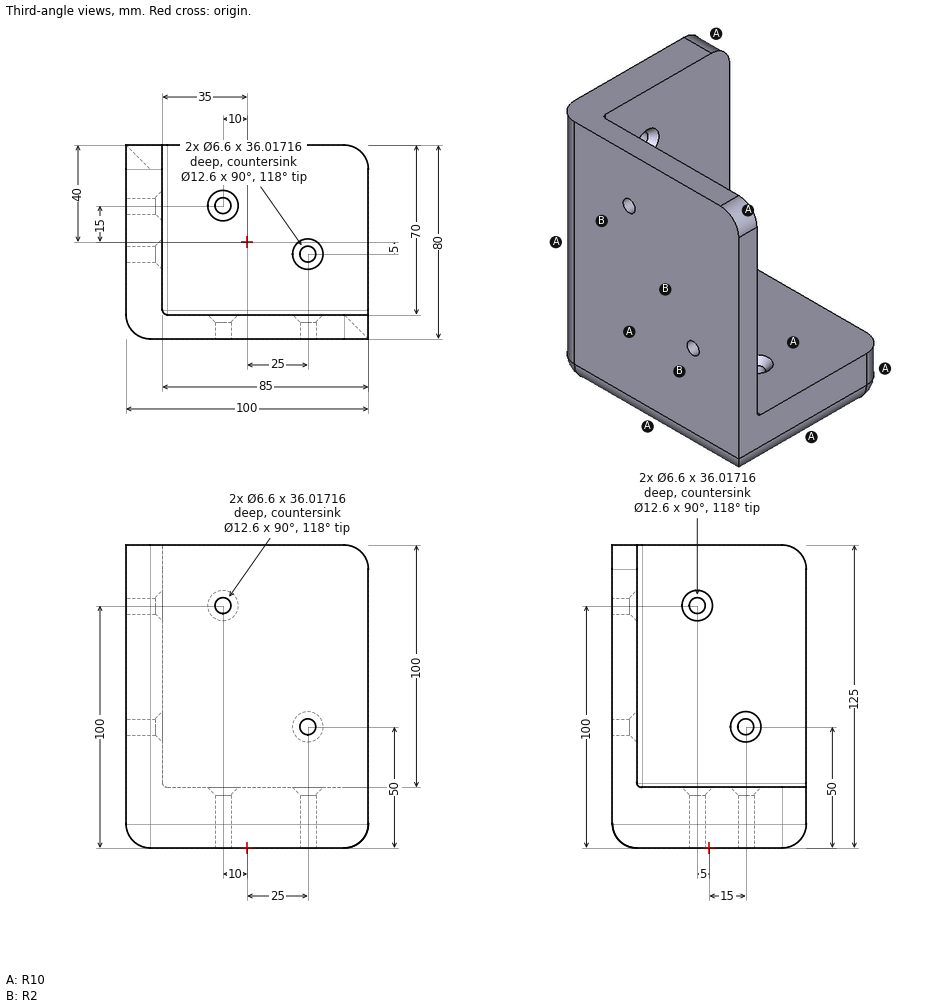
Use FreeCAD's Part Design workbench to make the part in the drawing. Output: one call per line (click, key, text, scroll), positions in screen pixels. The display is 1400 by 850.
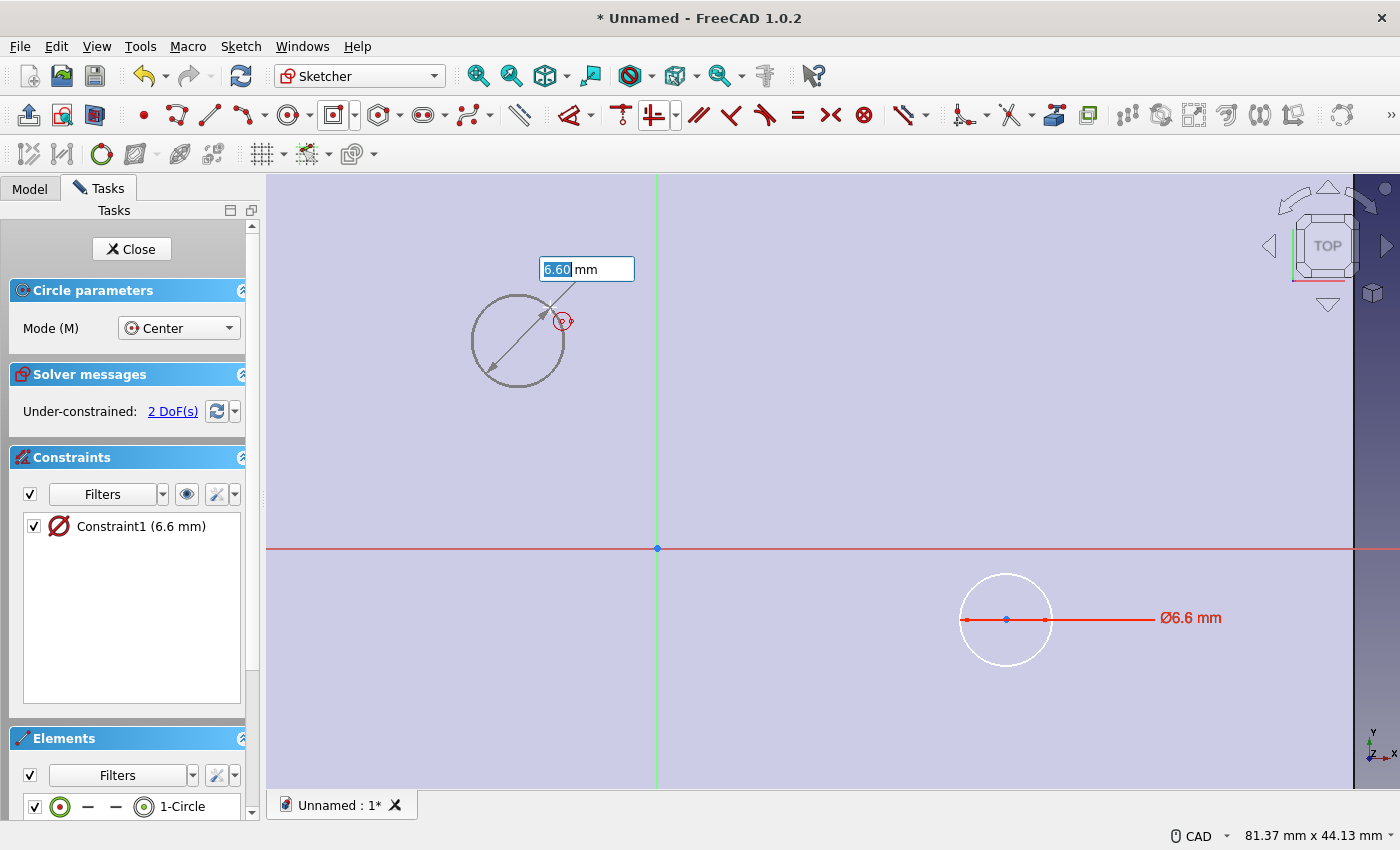
text(6.6)
key(Return)
key(Escape)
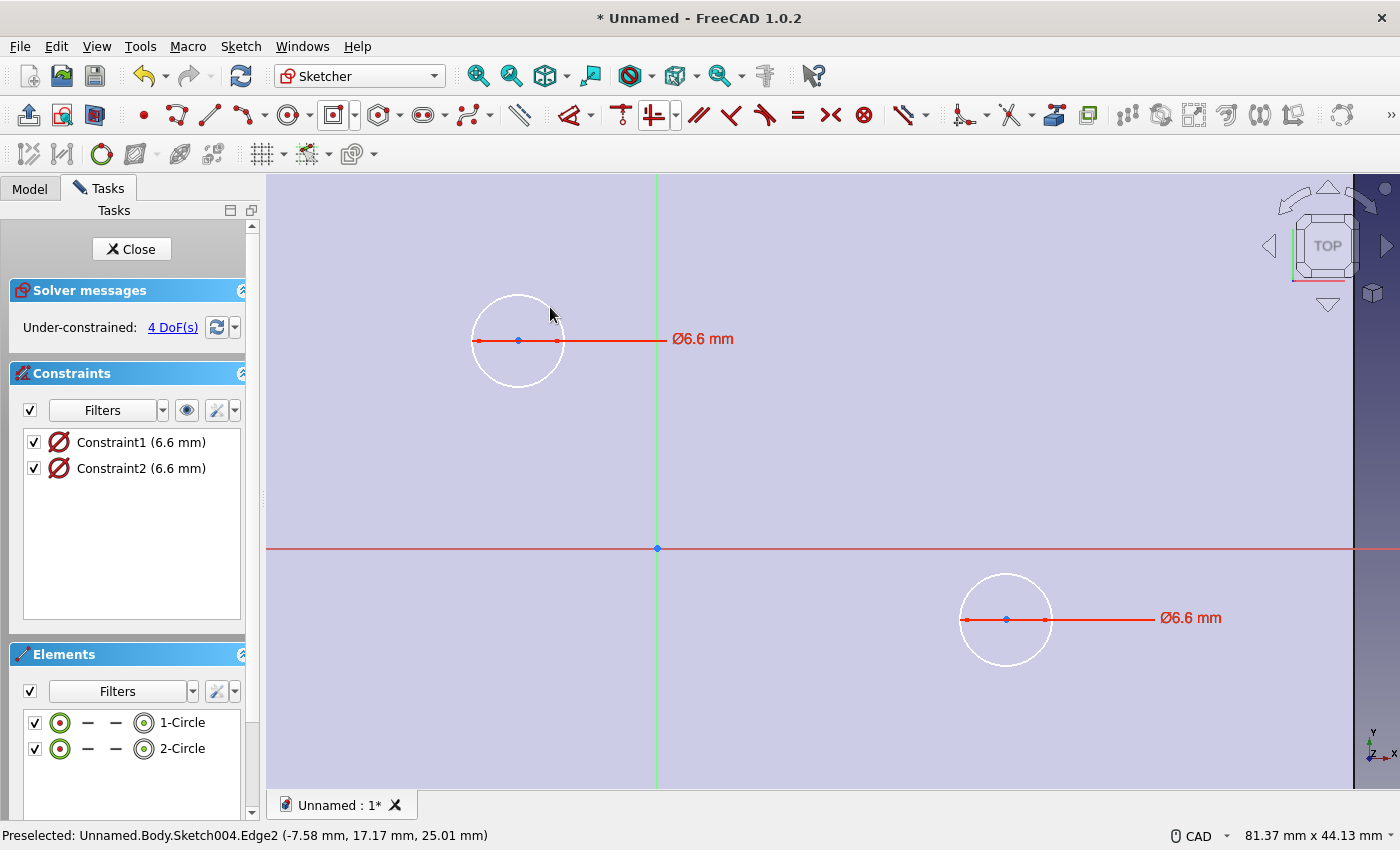
key(d)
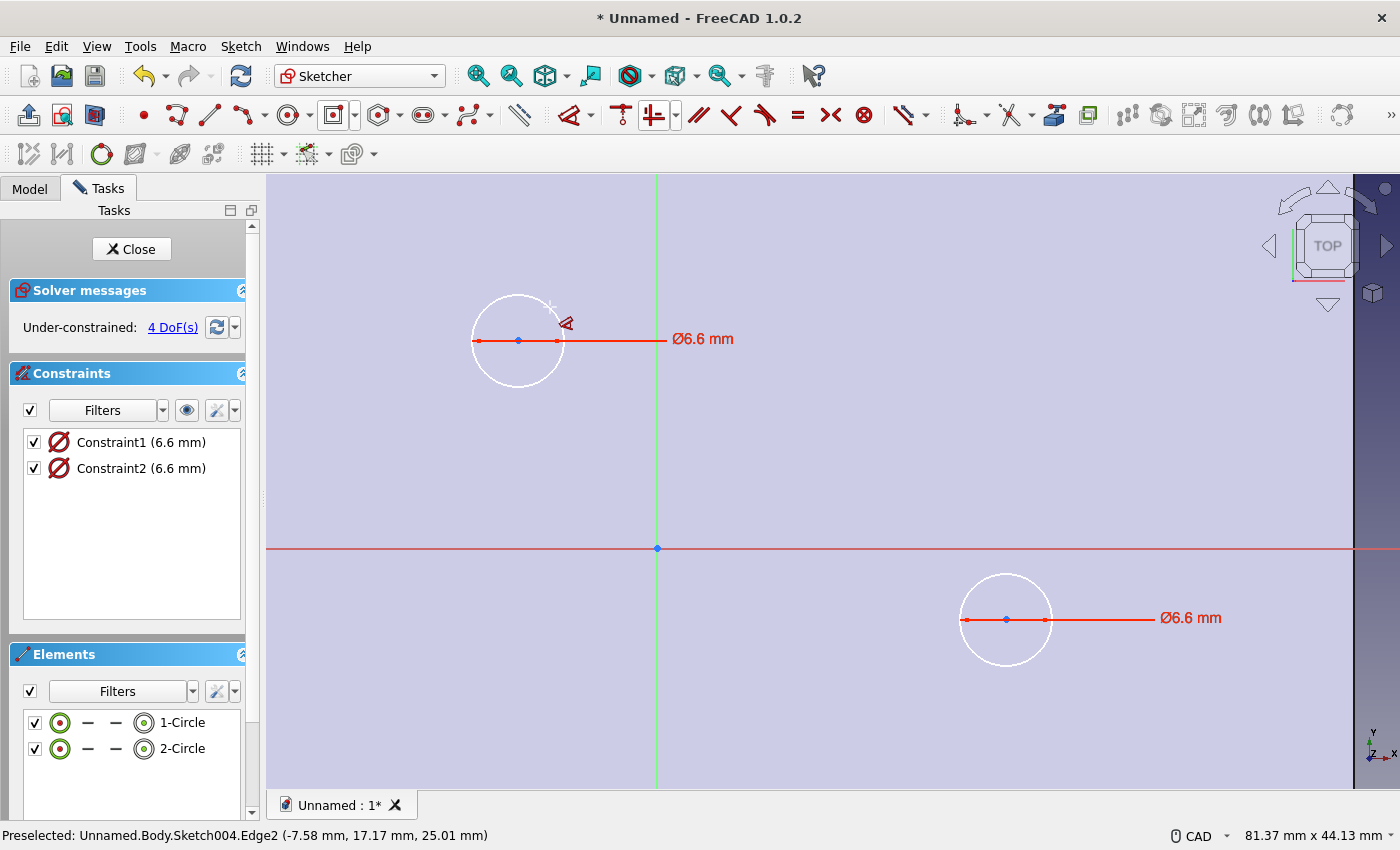
click(1006, 620)
click(1040, 568)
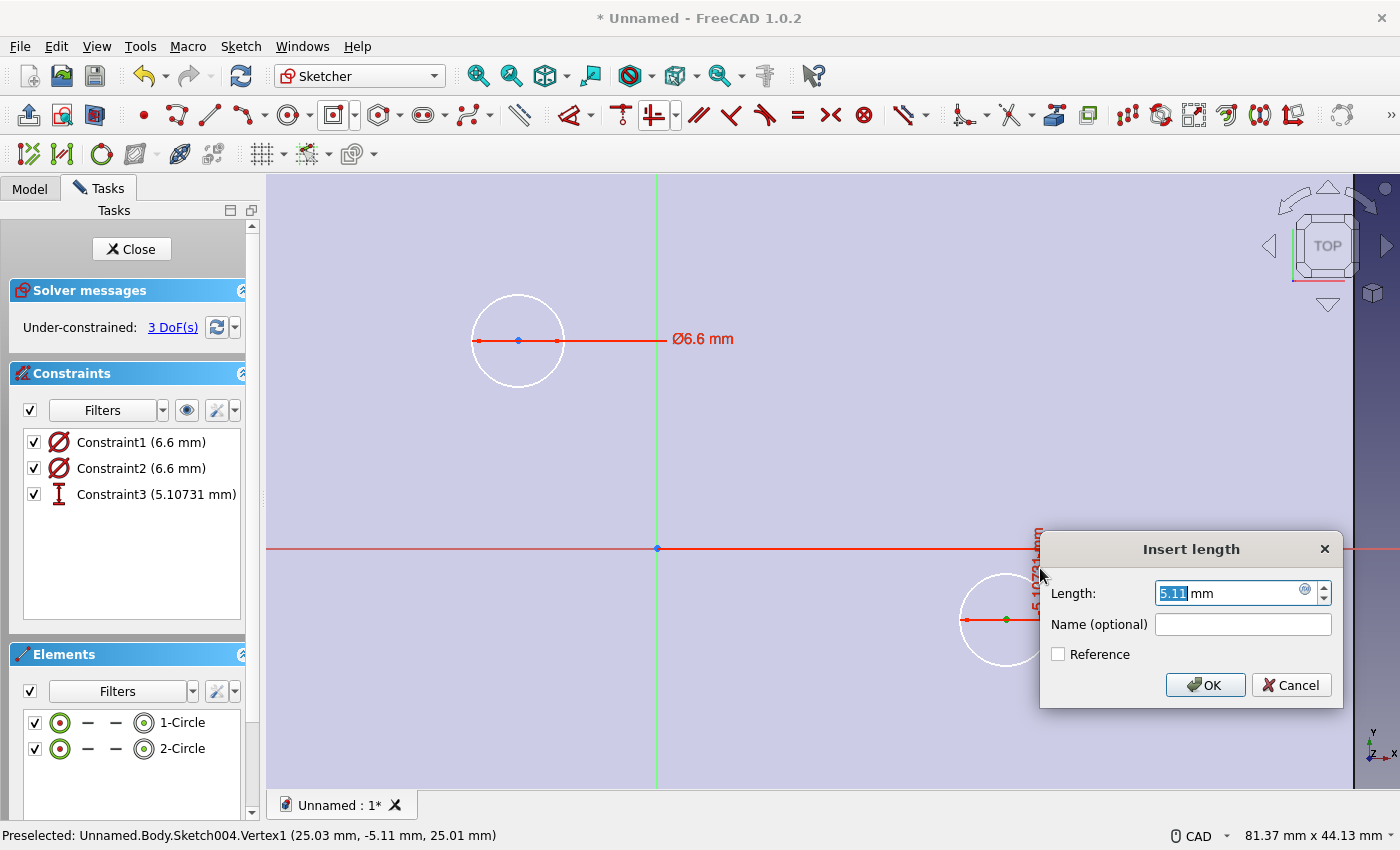
text(5)
key(Return)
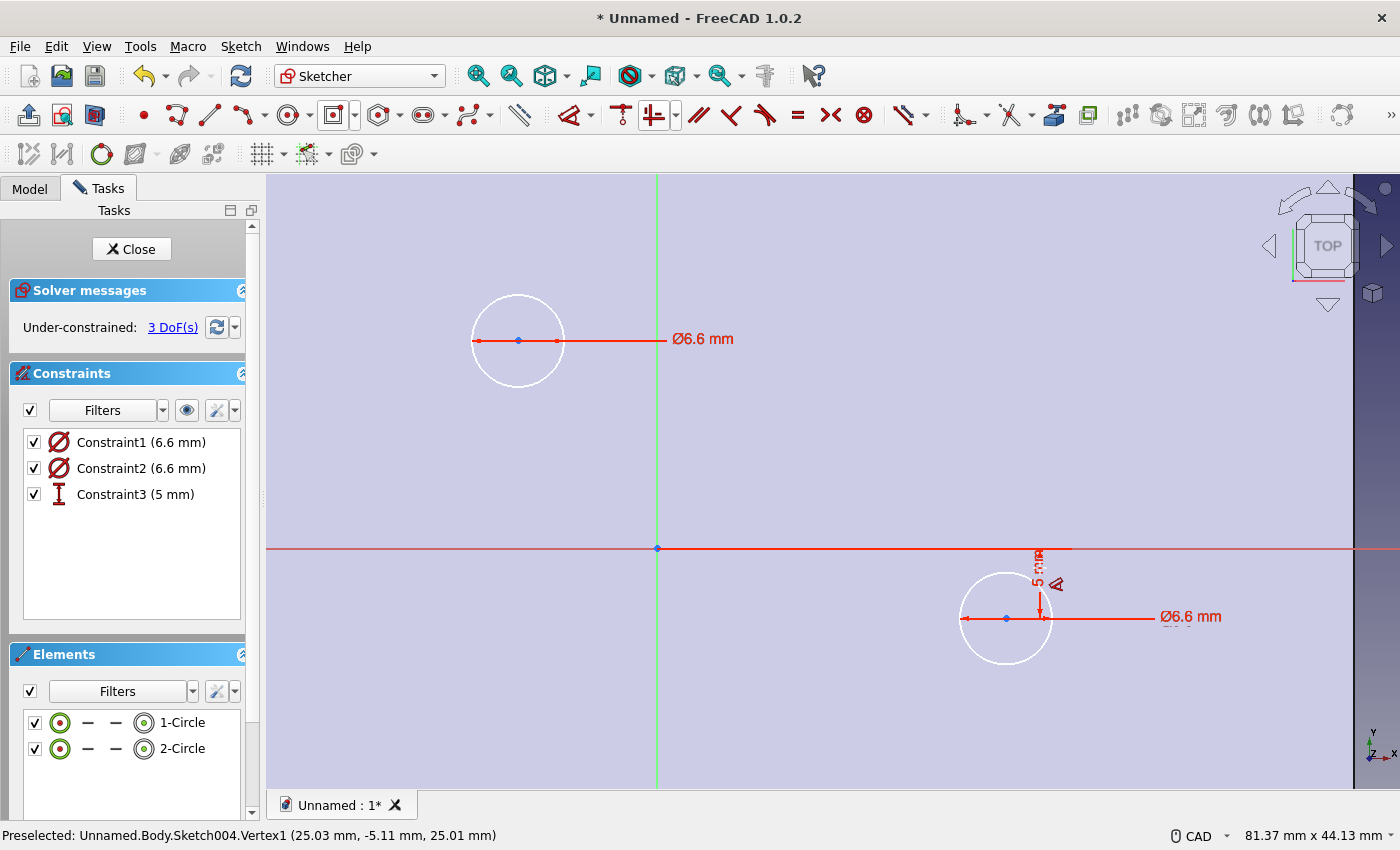
click(1006, 619)
click(832, 653)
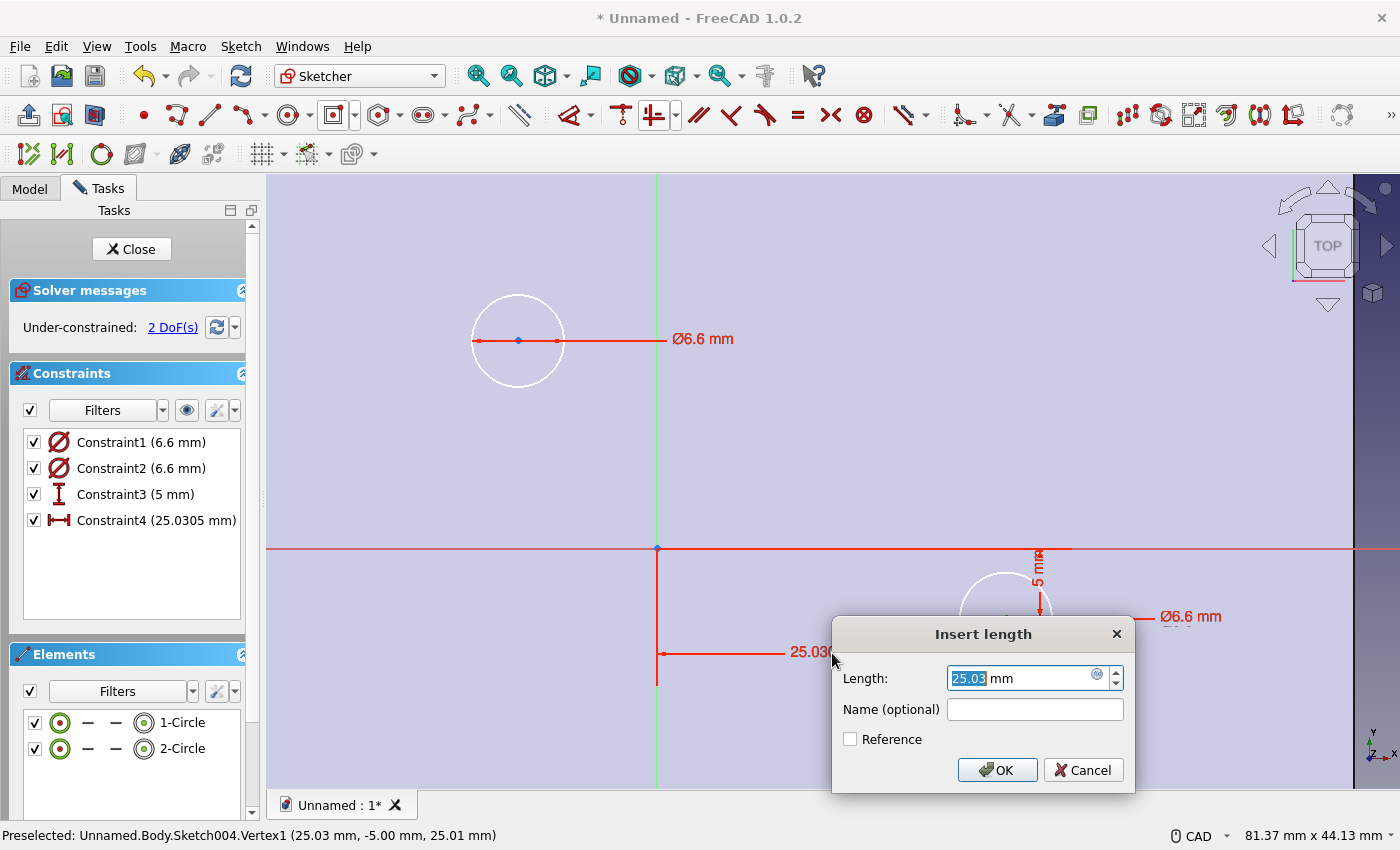
text(25)
key(Return)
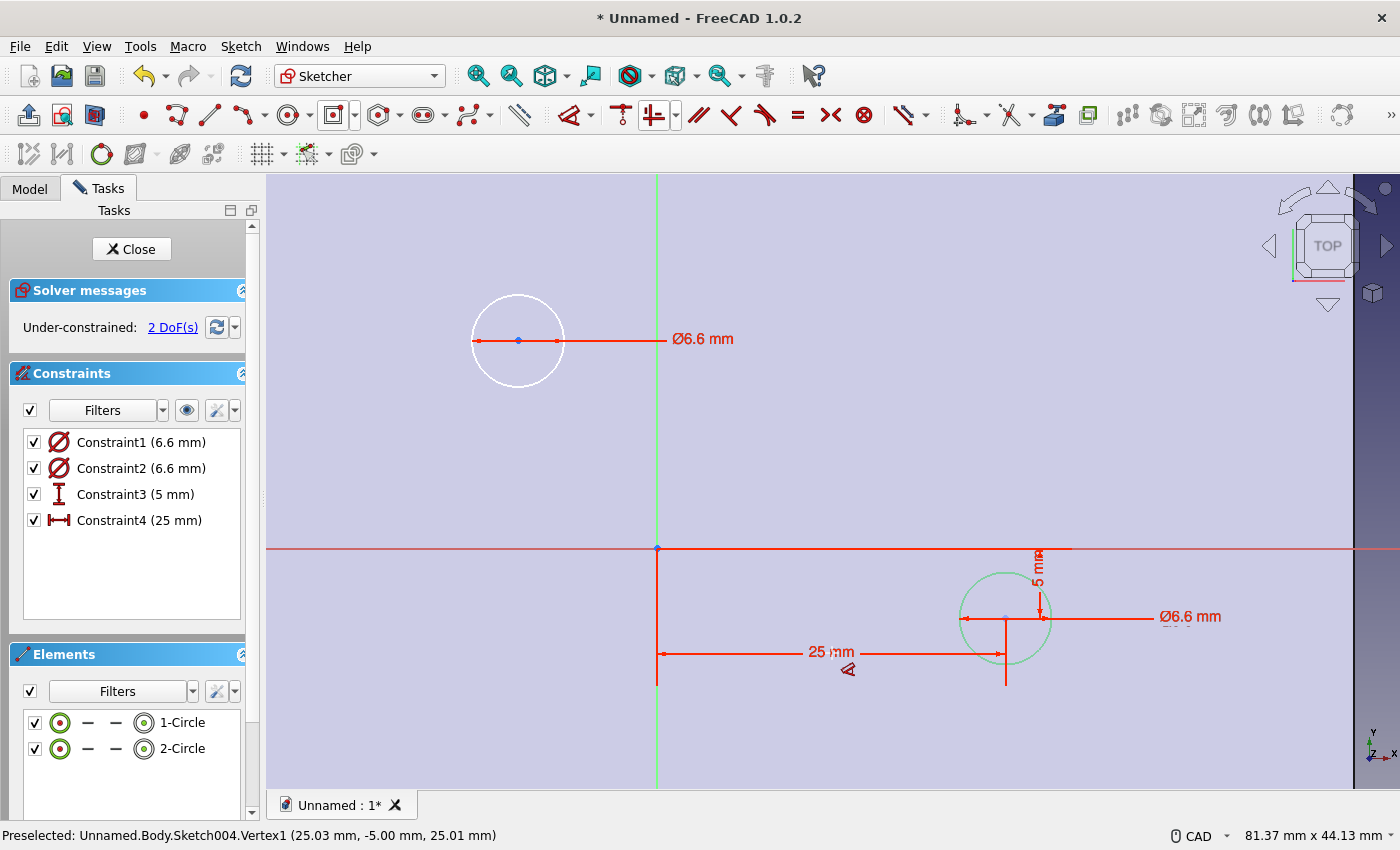
click(518, 341)
click(588, 307)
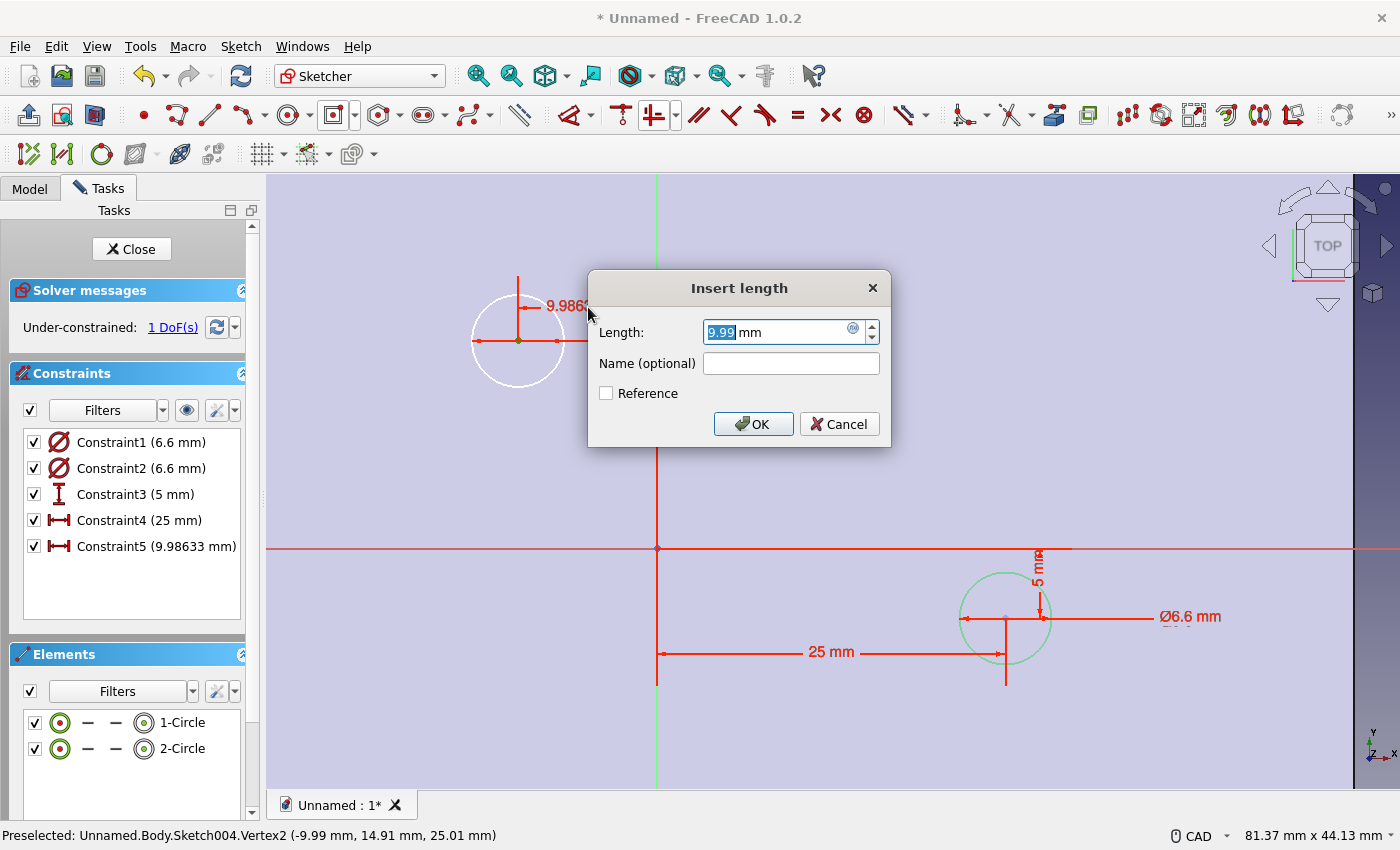
text(10)
key(Return)